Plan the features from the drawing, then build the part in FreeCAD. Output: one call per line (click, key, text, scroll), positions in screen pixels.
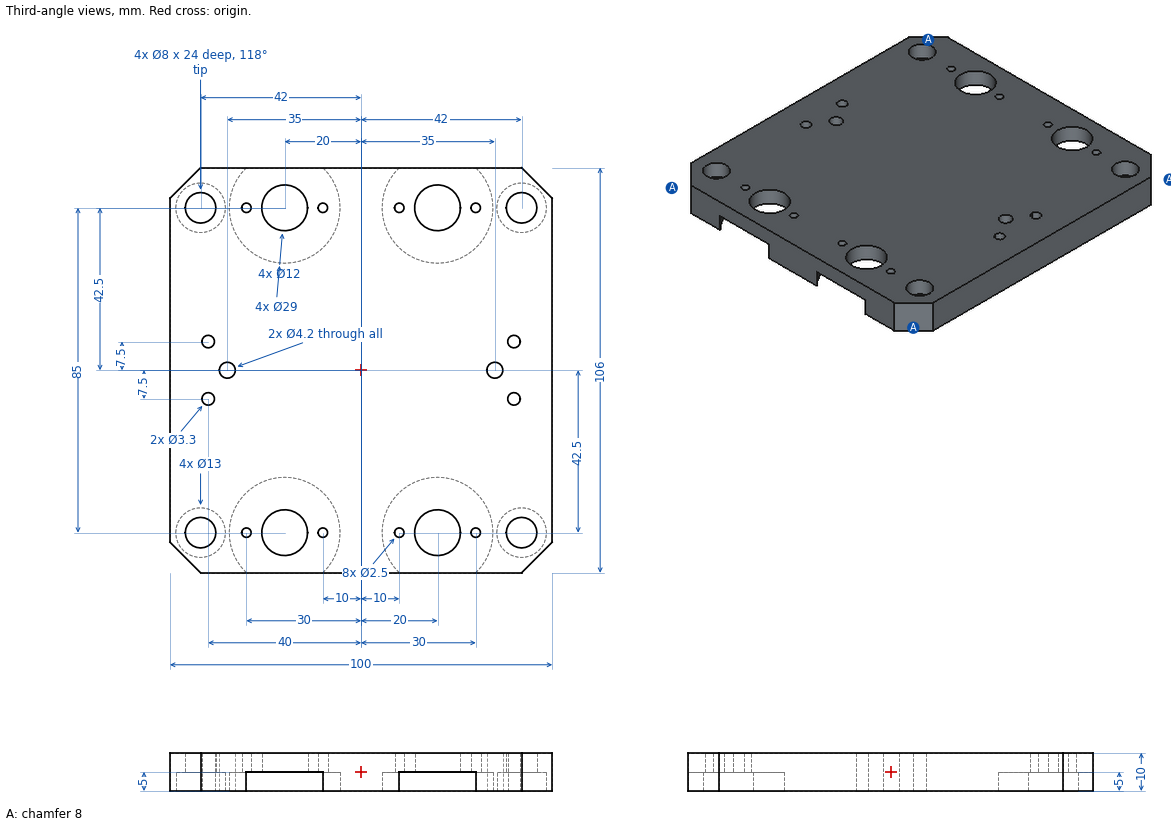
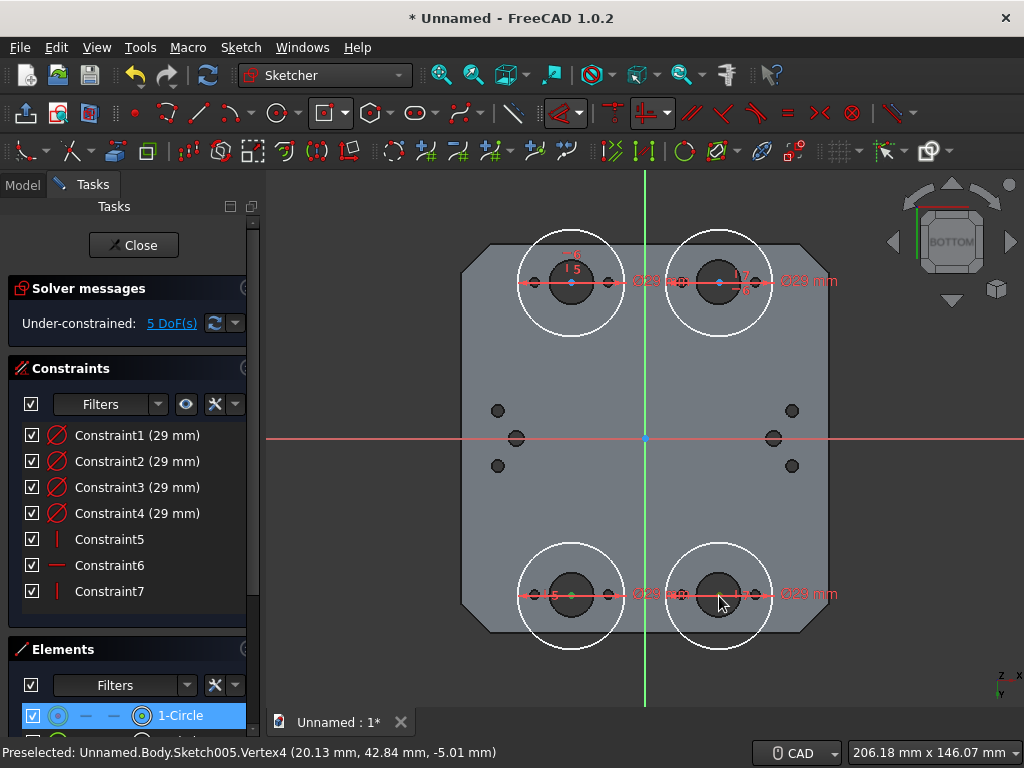
key(h)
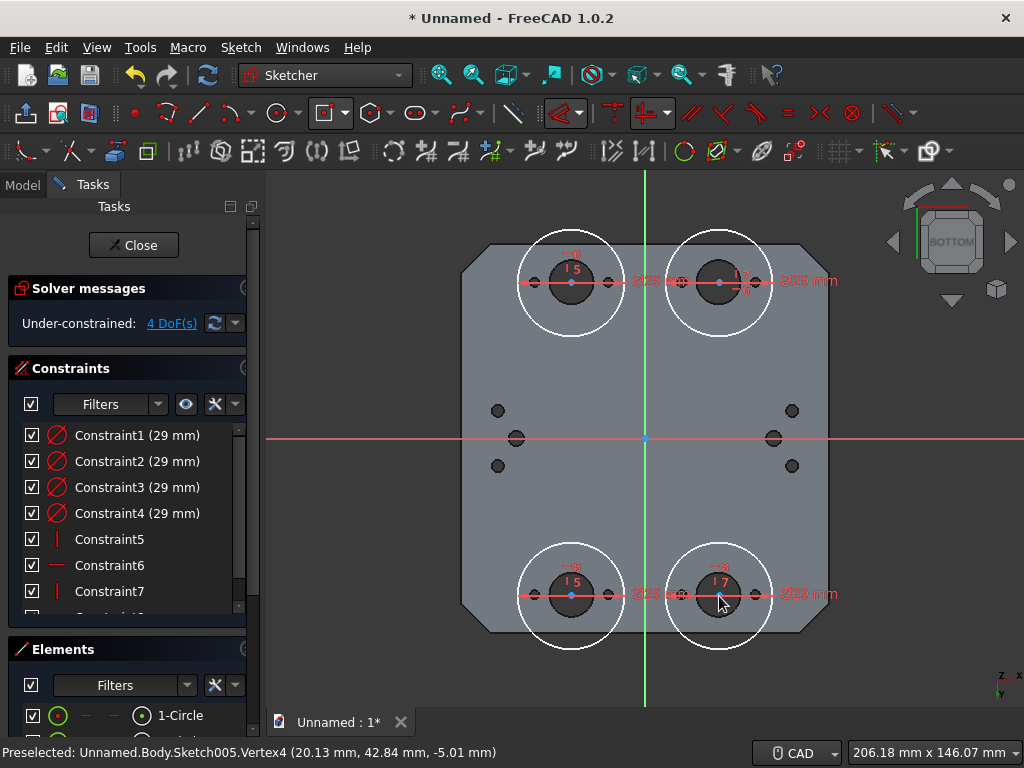
click(571, 596)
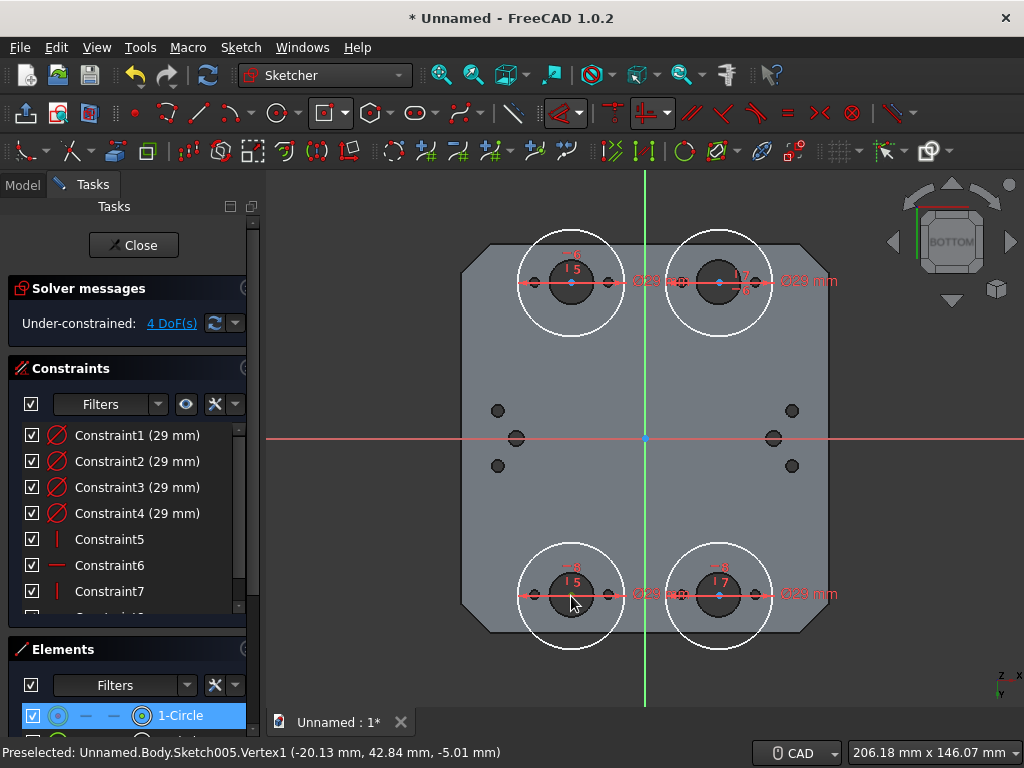
click(582, 114)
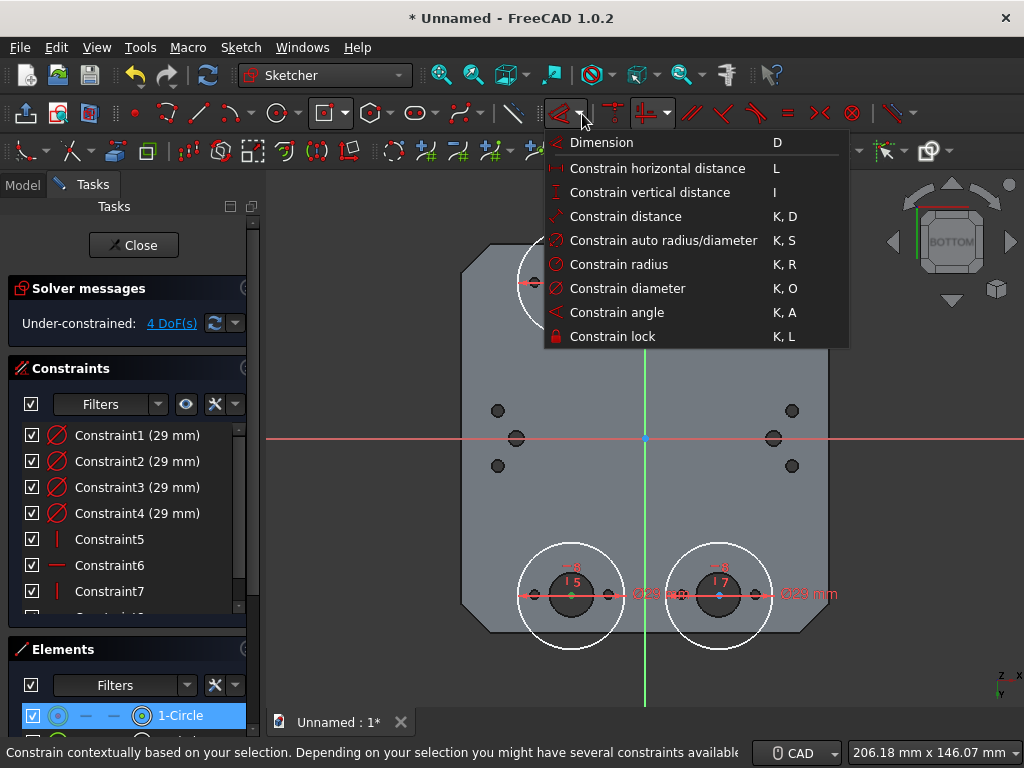
click(697, 168)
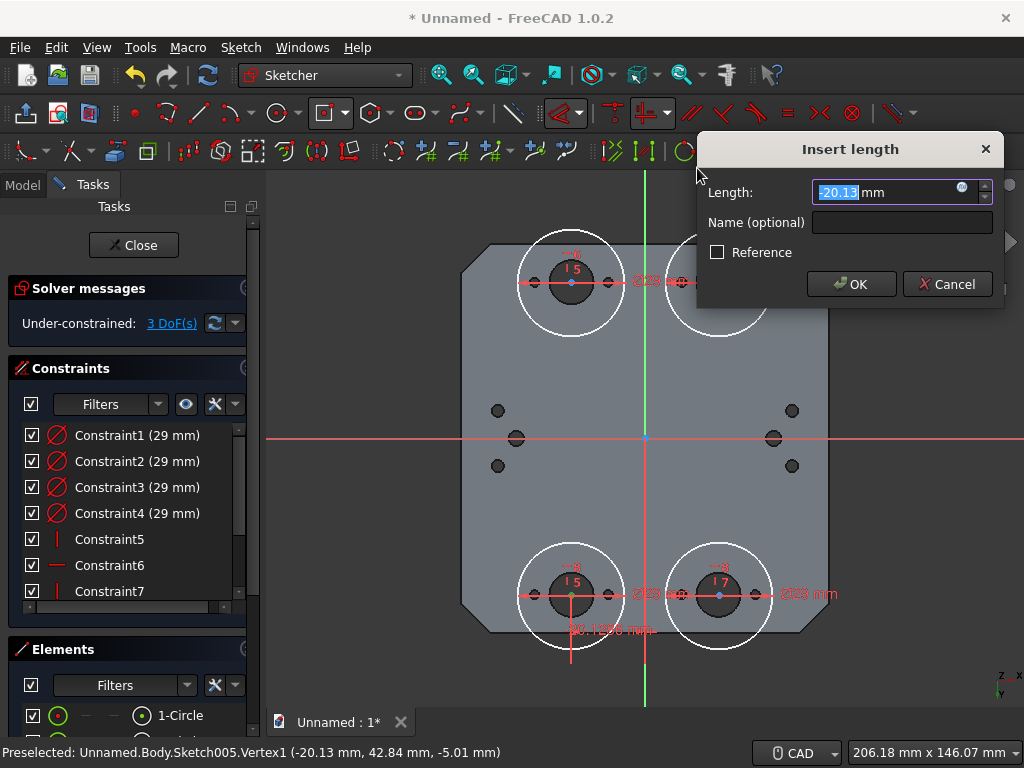
text(-20)
key(Return)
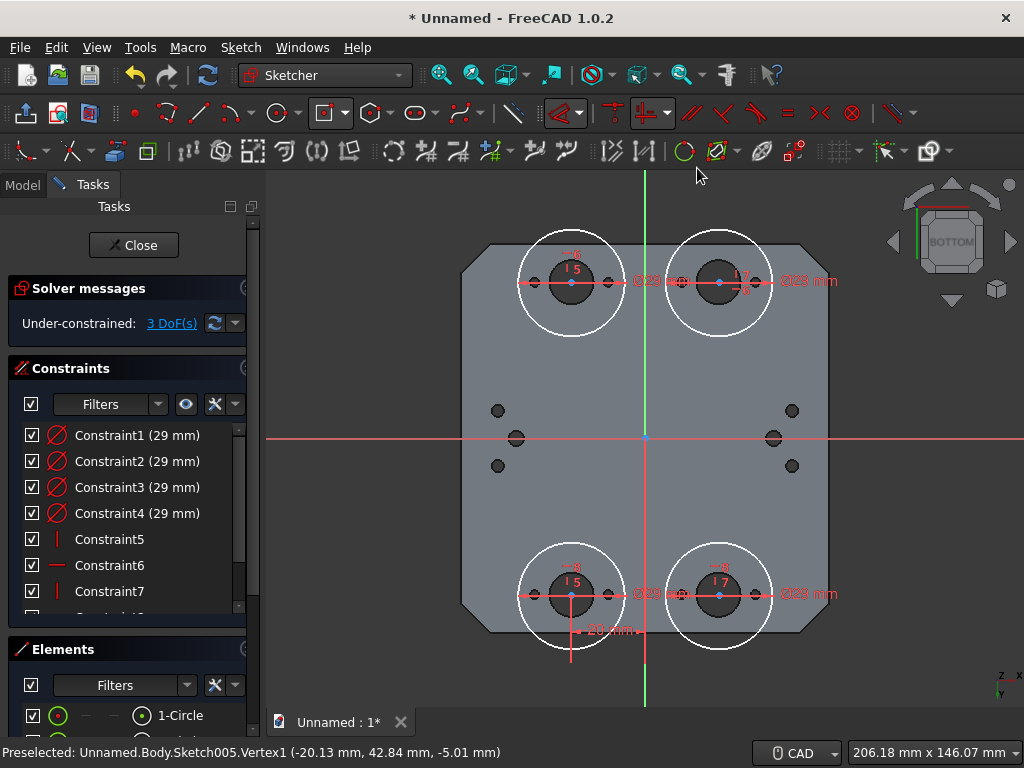
click(719, 283)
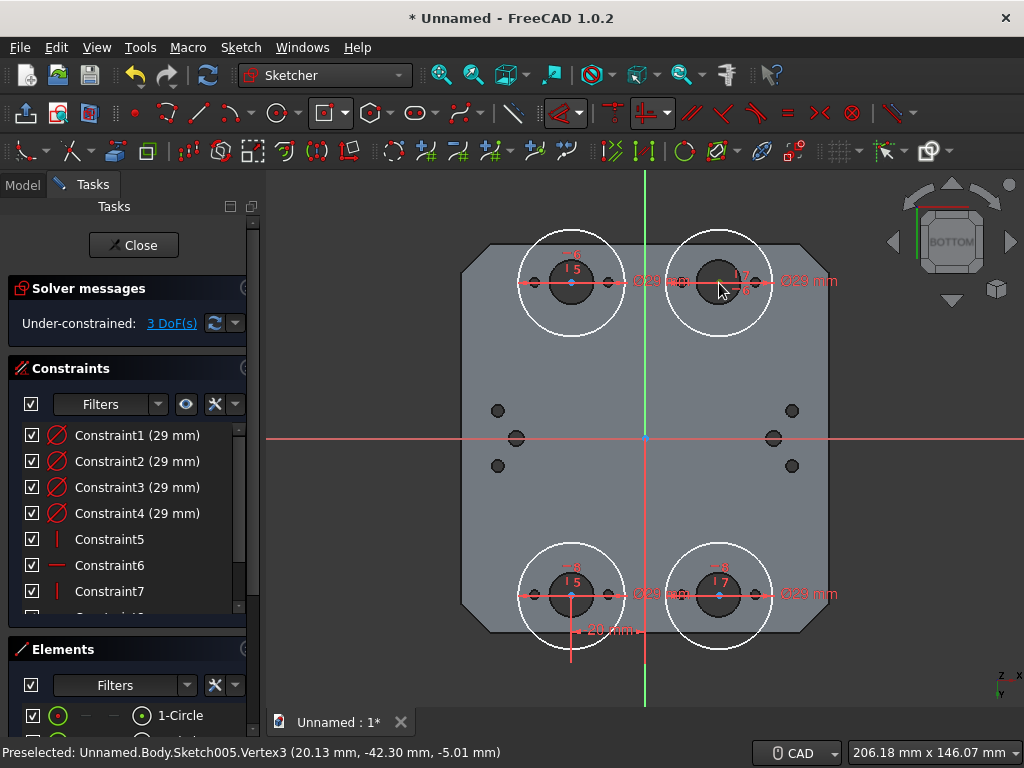
click(582, 114)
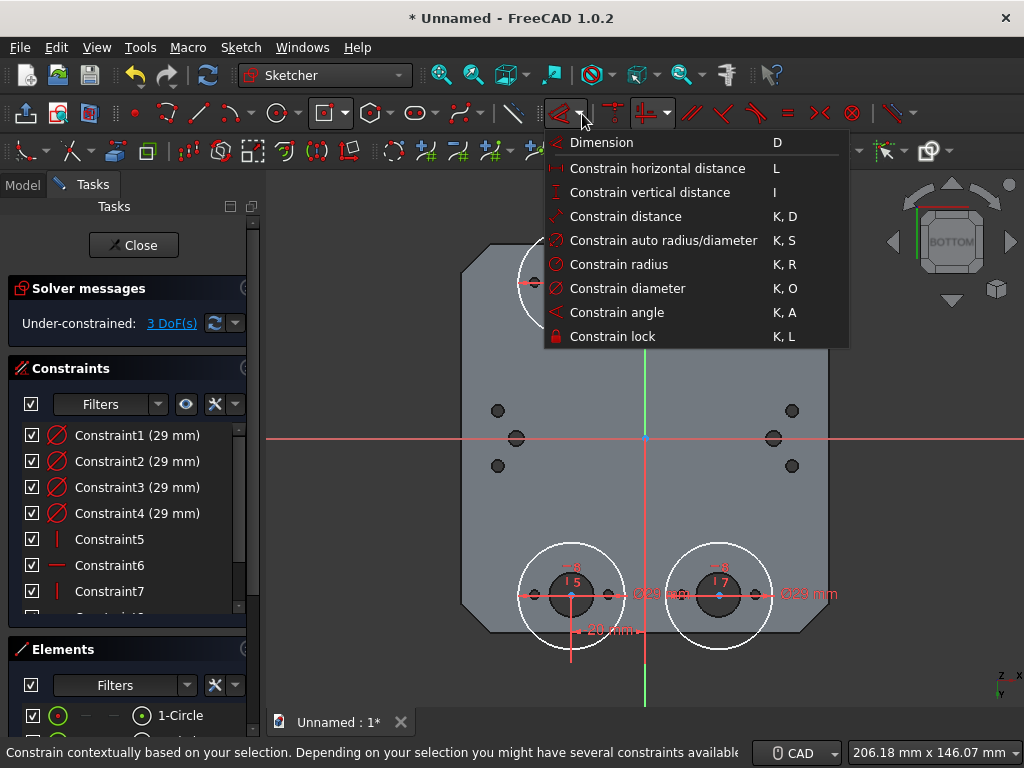
click(697, 168)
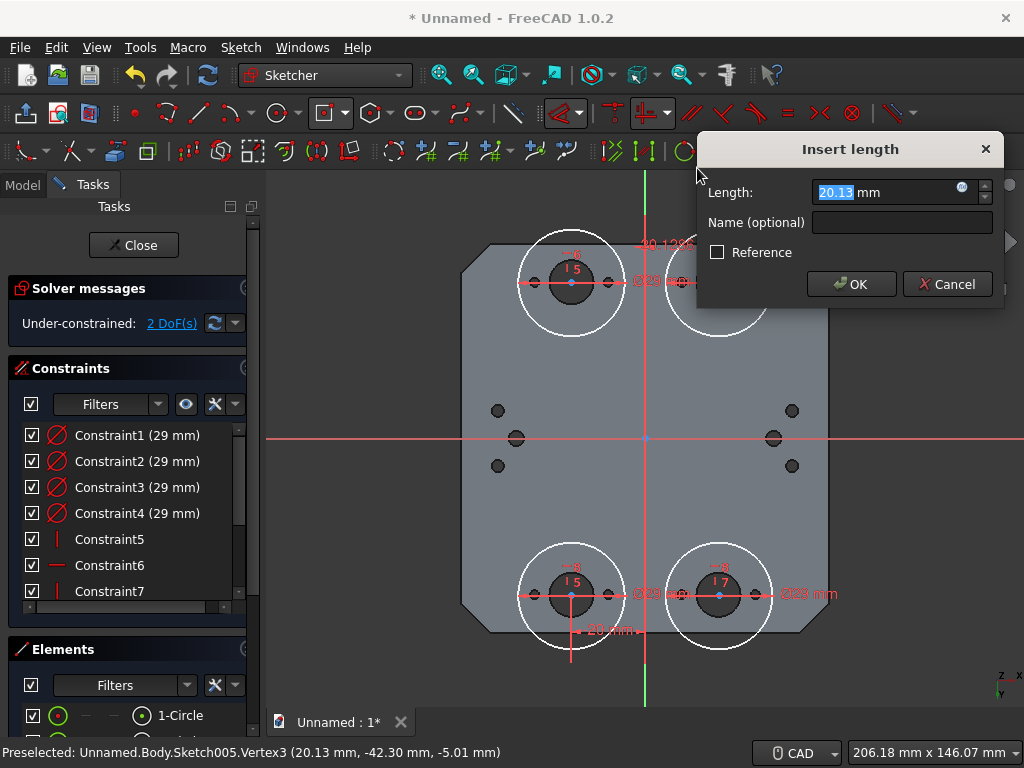
text(20)
key(Return)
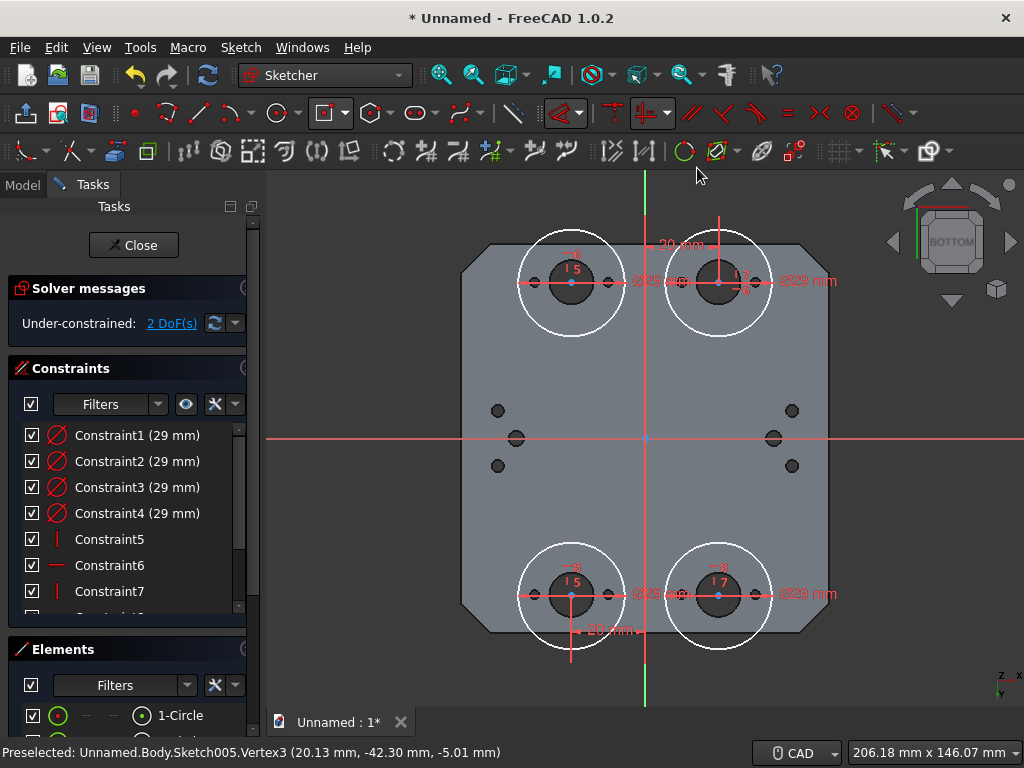
click(571, 596)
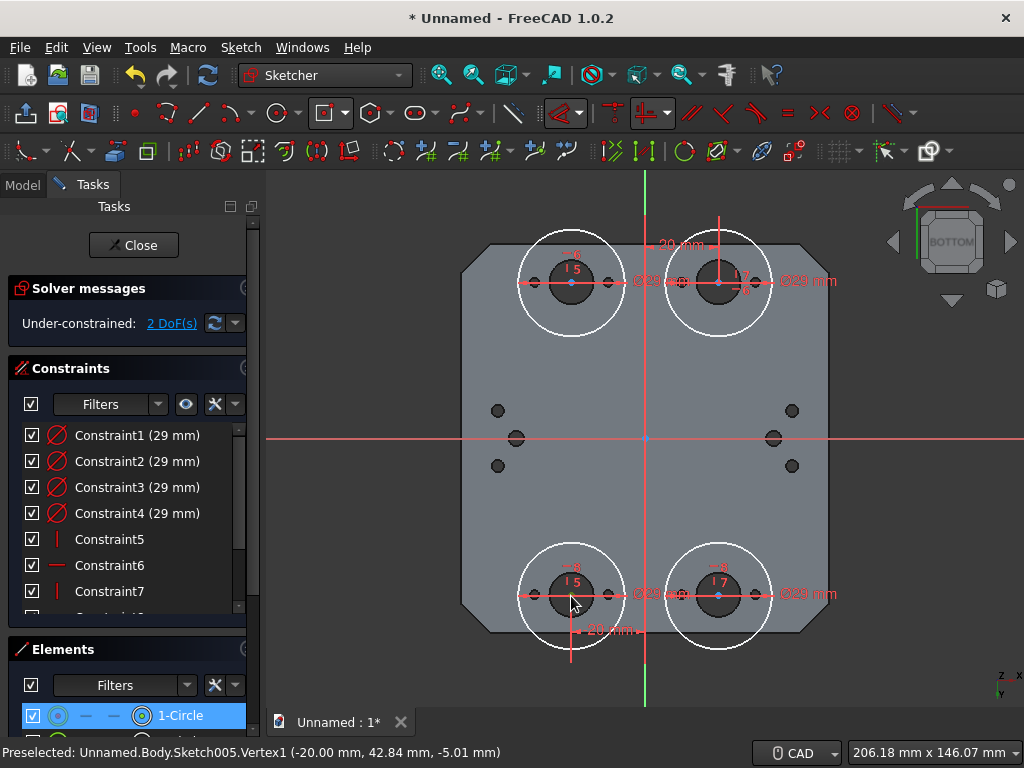
click(571, 283)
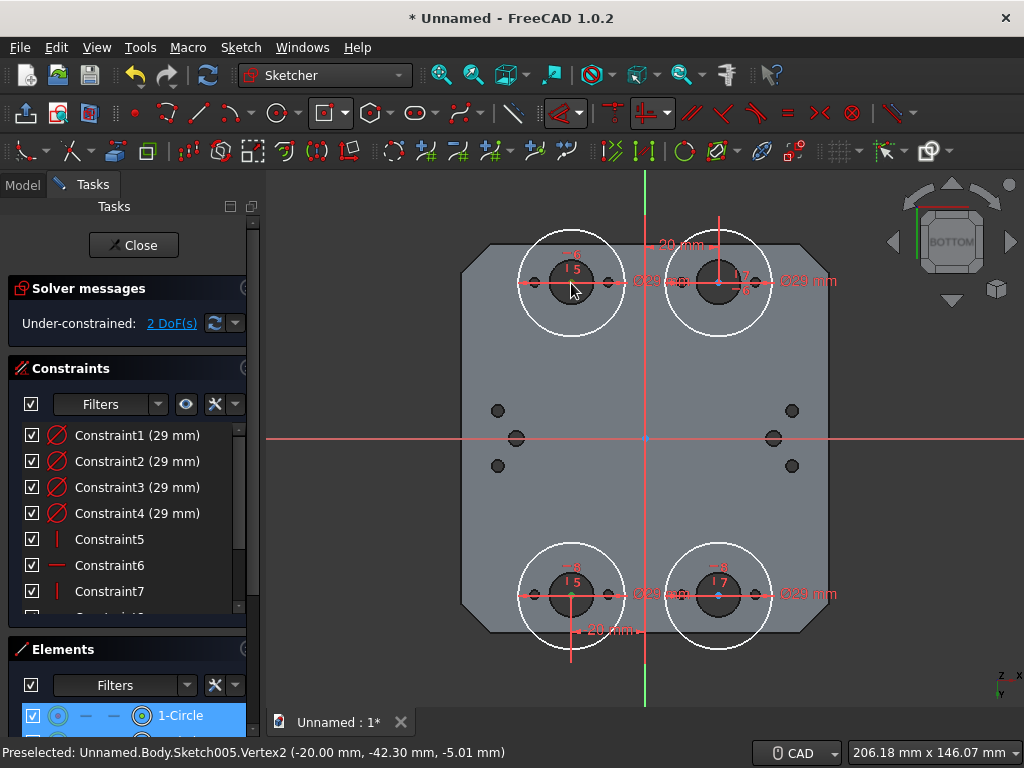
click(582, 114)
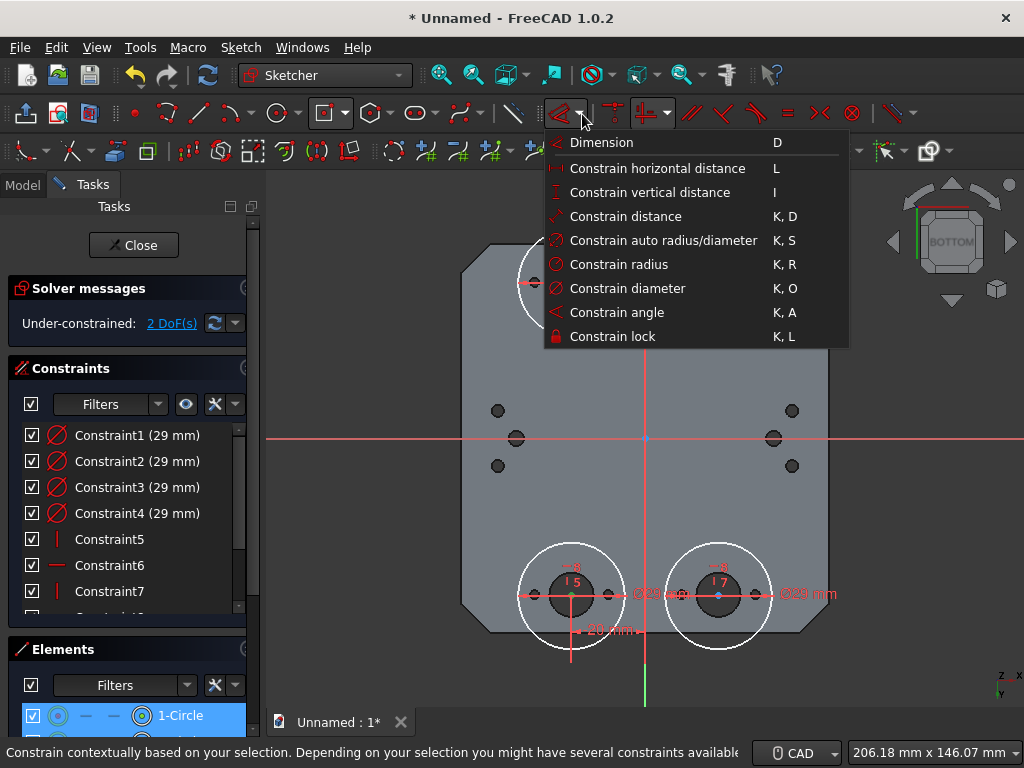
click(697, 192)